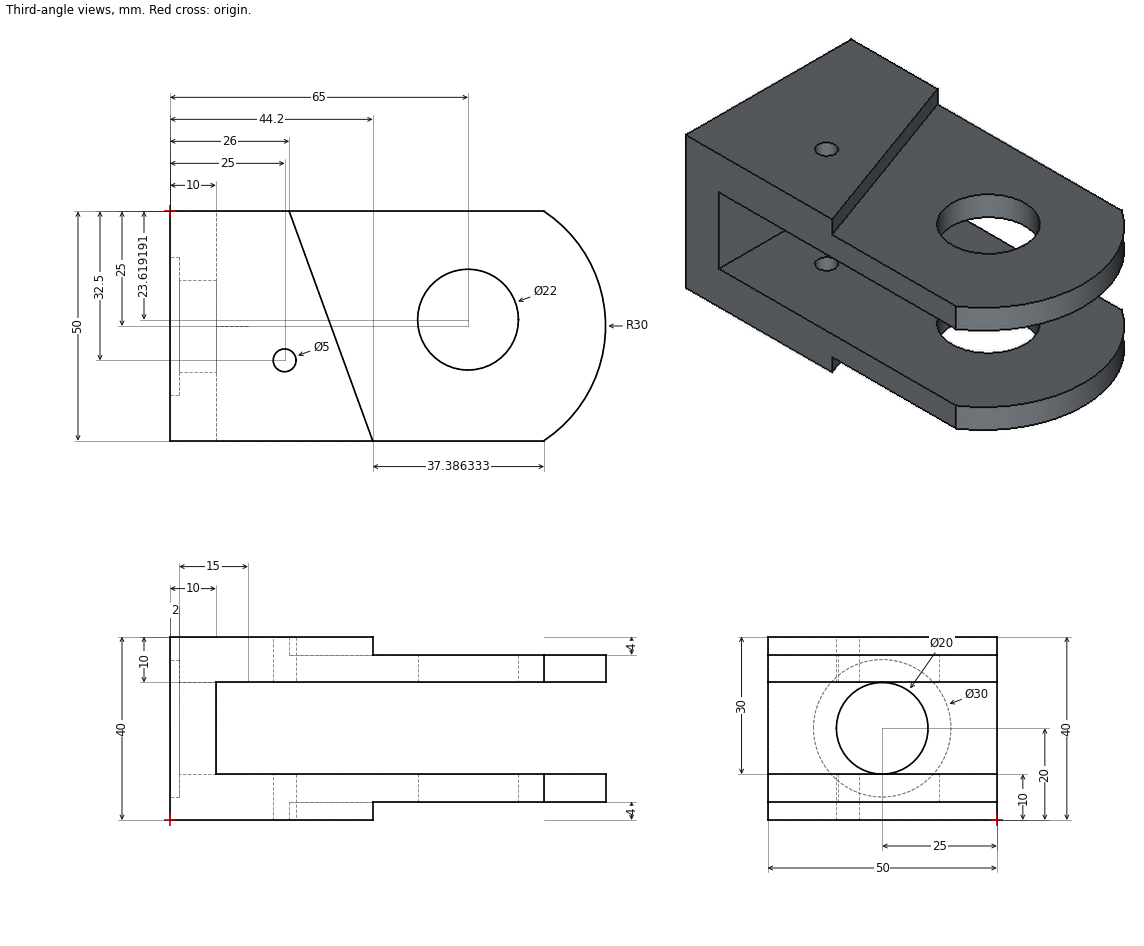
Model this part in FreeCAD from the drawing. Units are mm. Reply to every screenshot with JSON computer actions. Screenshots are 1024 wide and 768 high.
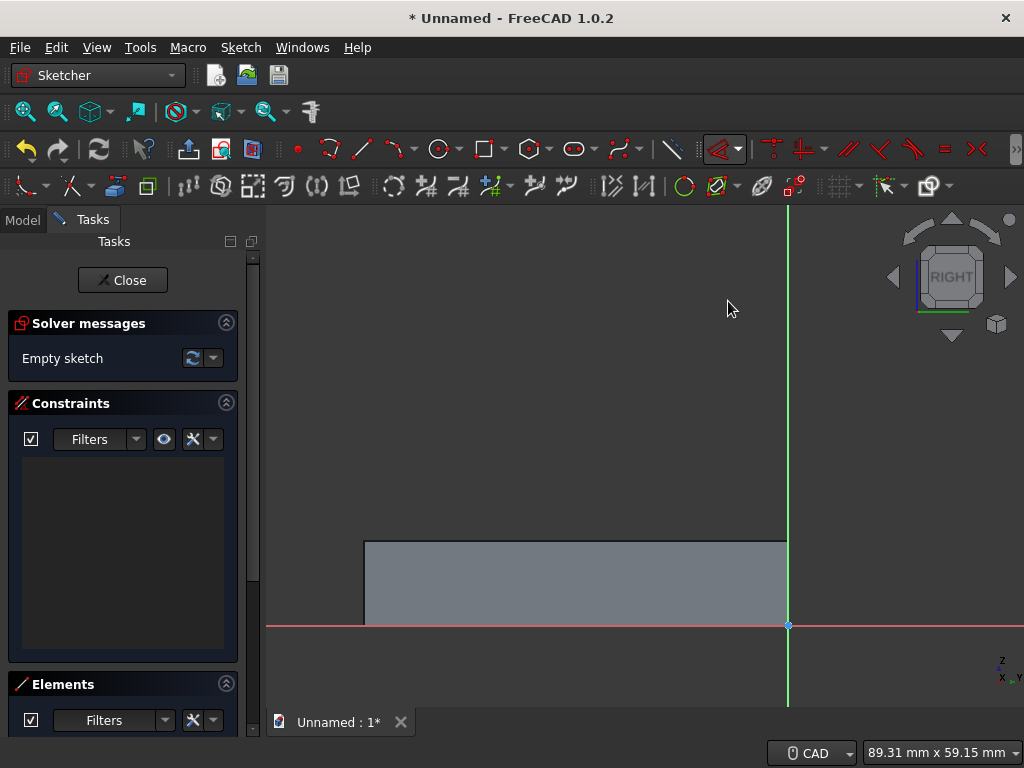
{"action": "left_click", "coordinate": [484, 150]}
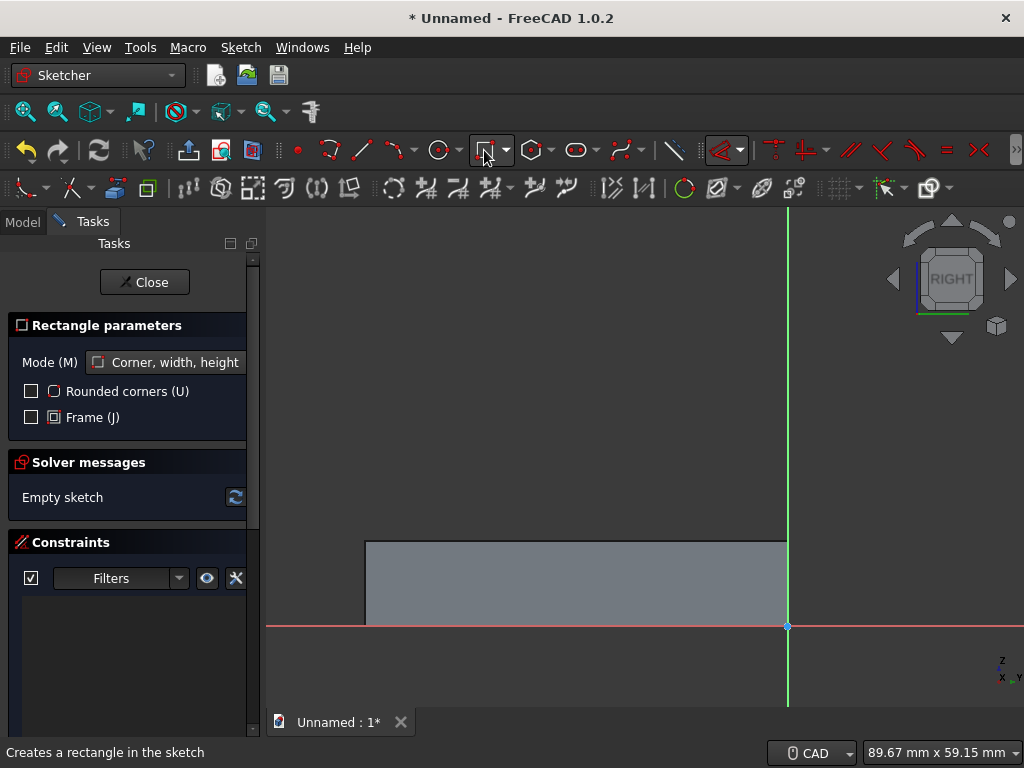
{"action": "left_click", "coordinate": [365, 288]}
{"action": "left_click", "coordinate": [788, 541]}
{"action": "key", "text": "Escape"}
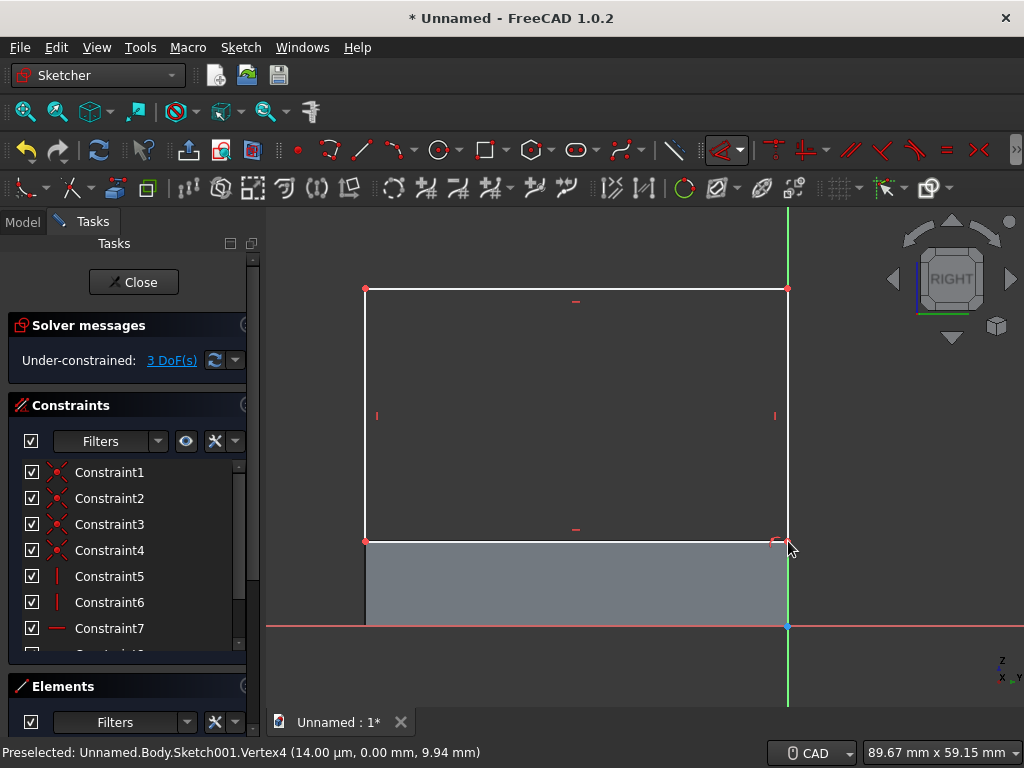
{"action": "left_click", "coordinate": [365, 365]}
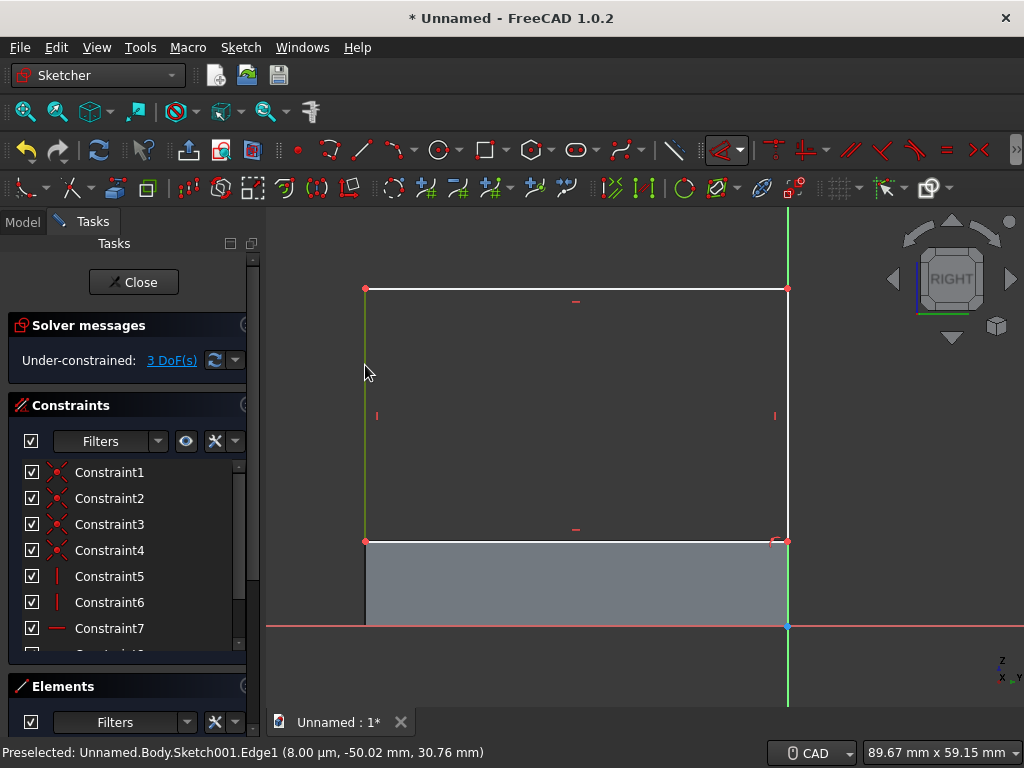
{"action": "key", "text": "i"}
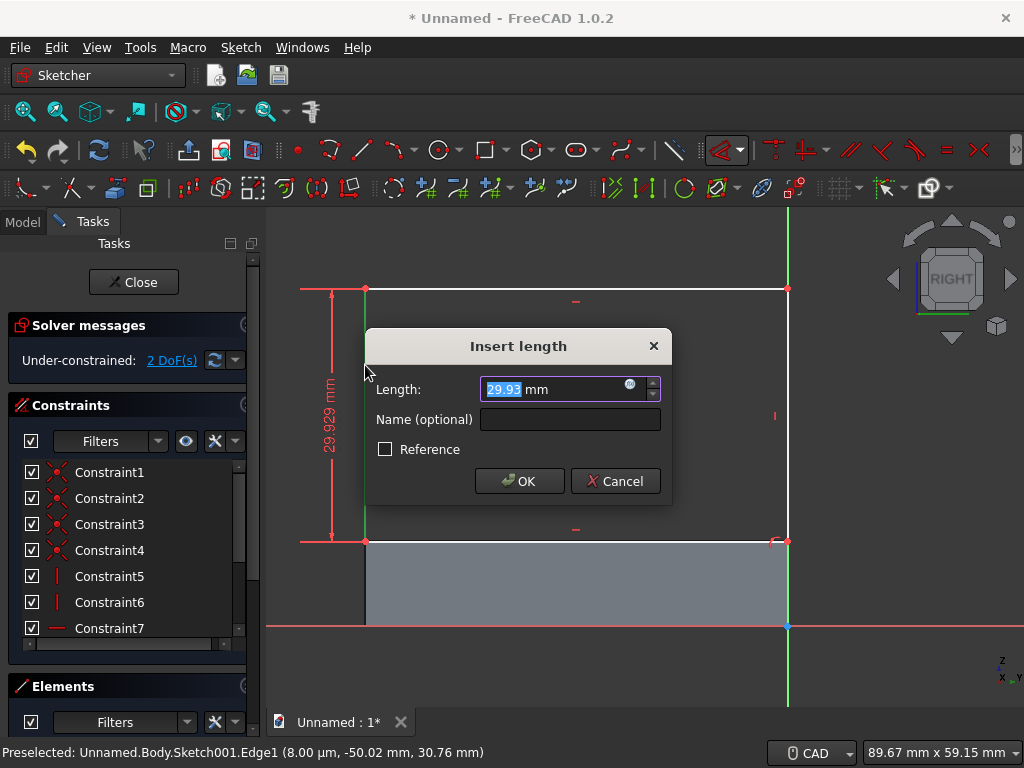
{"action": "type", "text": "30"}
{"action": "key", "text": "Return"}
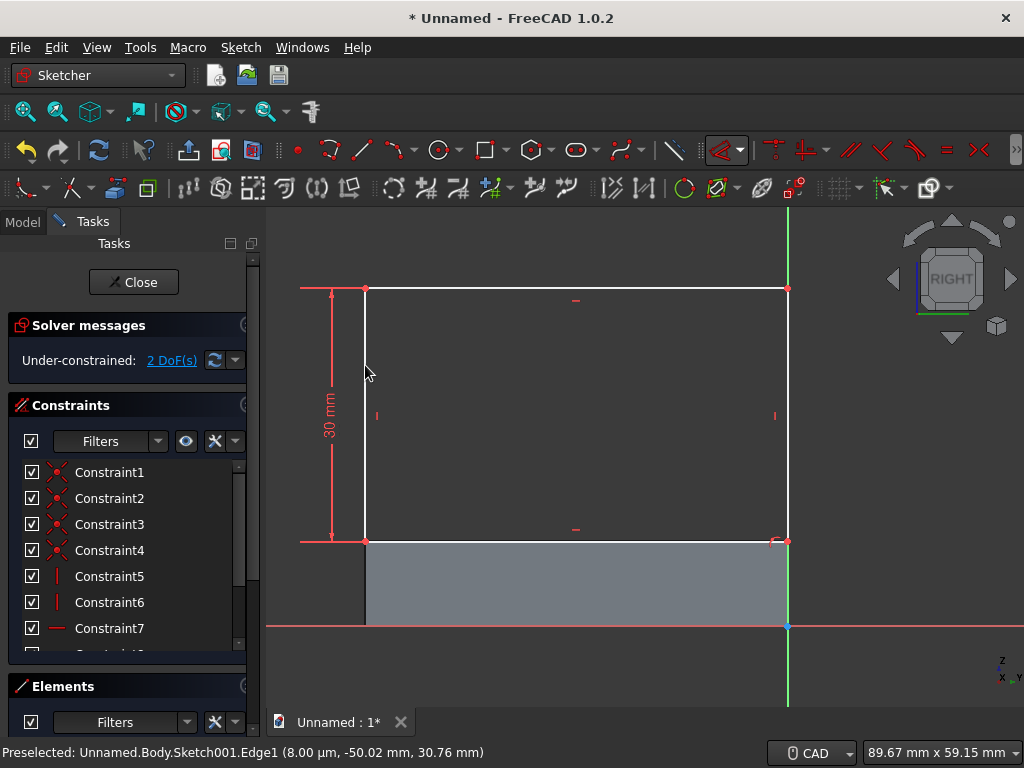
{"action": "left_click", "coordinate": [492, 542]}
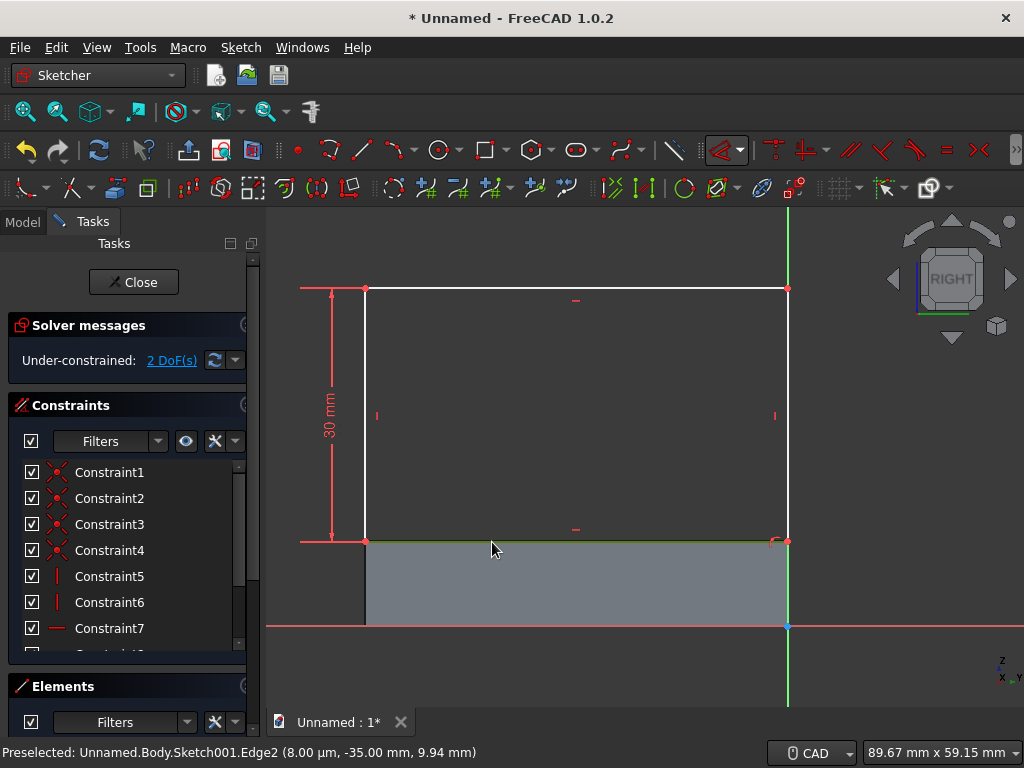
{"action": "left_click", "coordinate": [742, 150]}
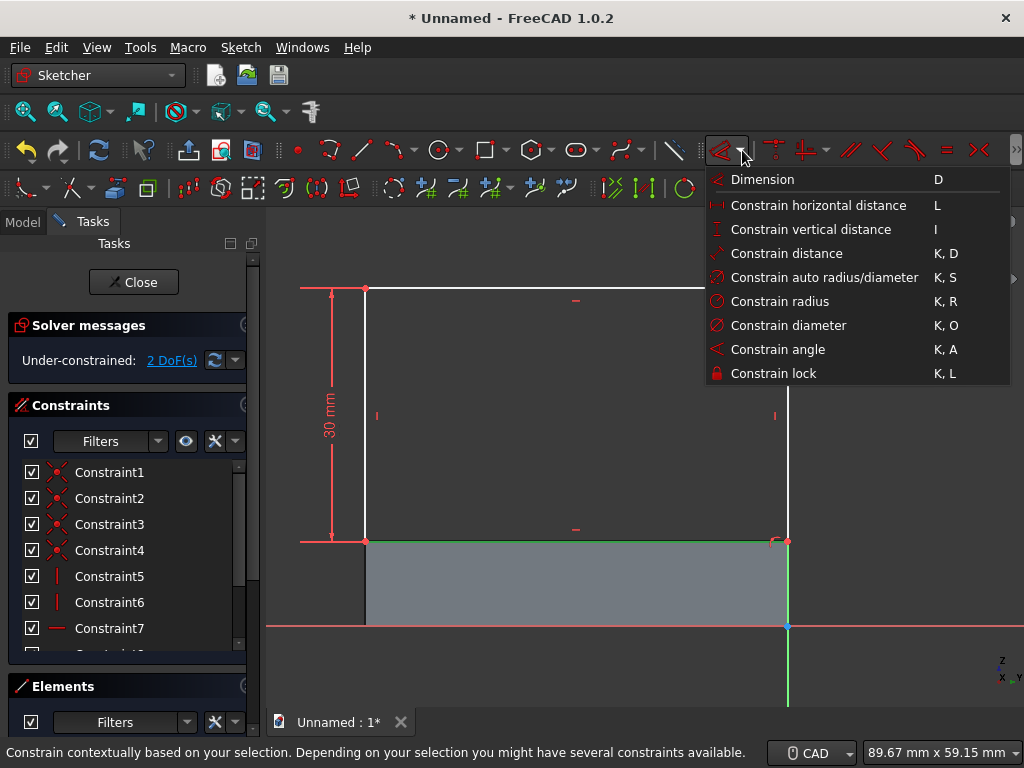
{"action": "left_click", "coordinate": [858, 205]}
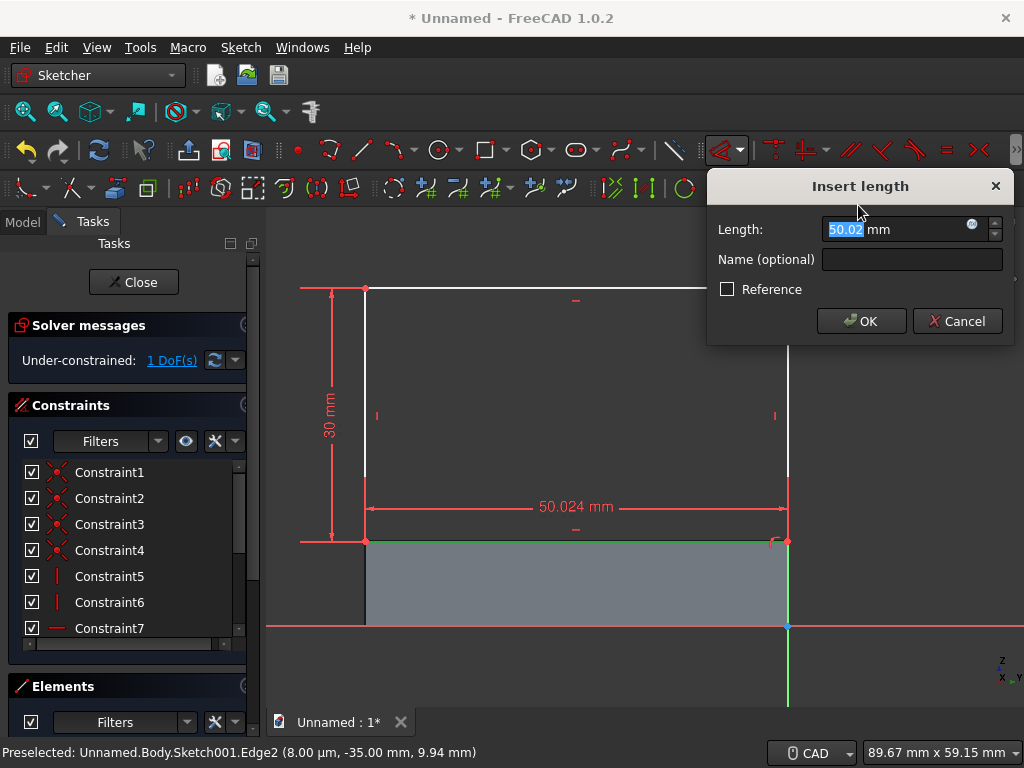
{"action": "type", "text": "50"}
{"action": "key", "text": "Return"}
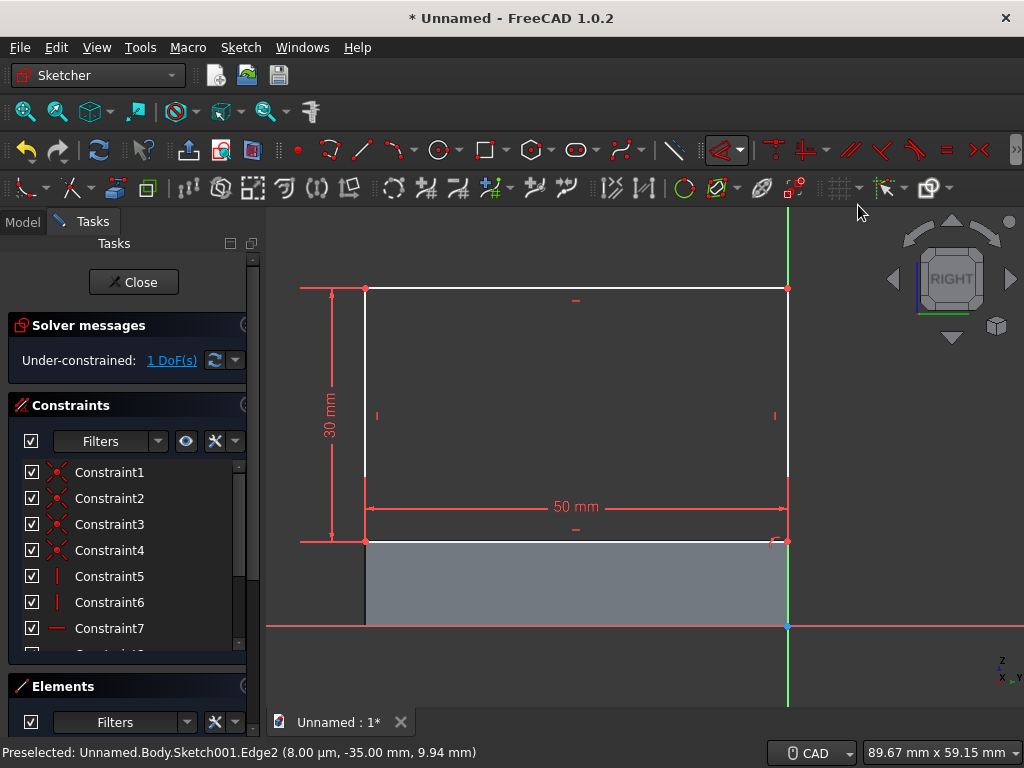
{"action": "left_click", "coordinate": [365, 288]}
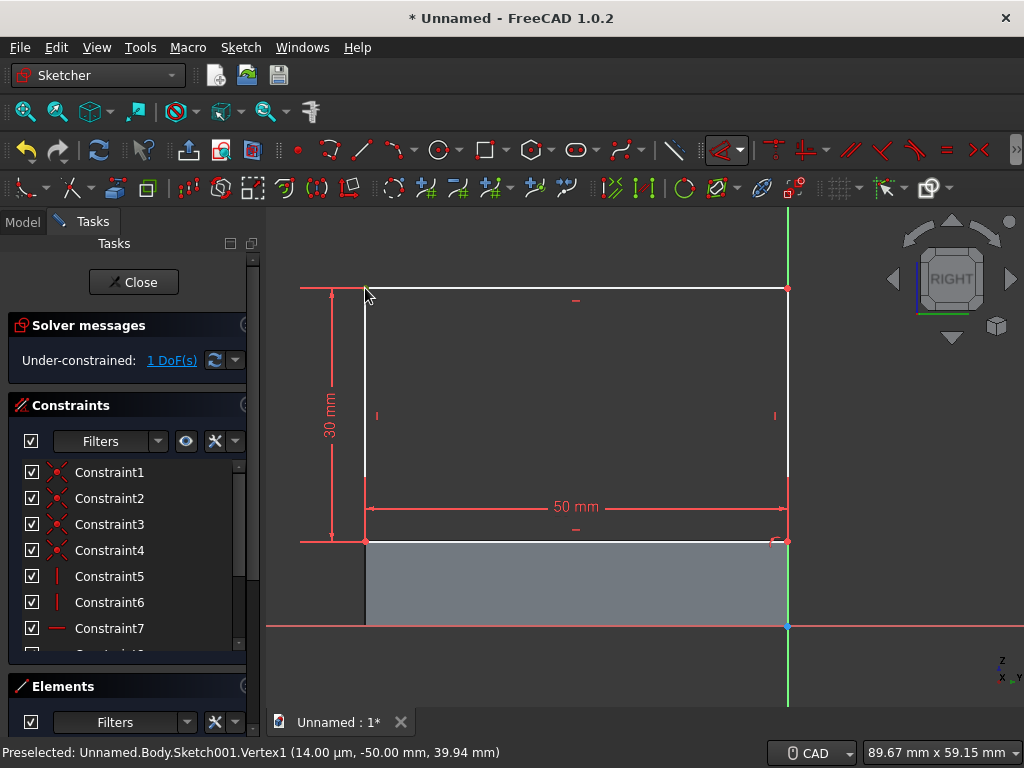
{"action": "key", "text": "i"}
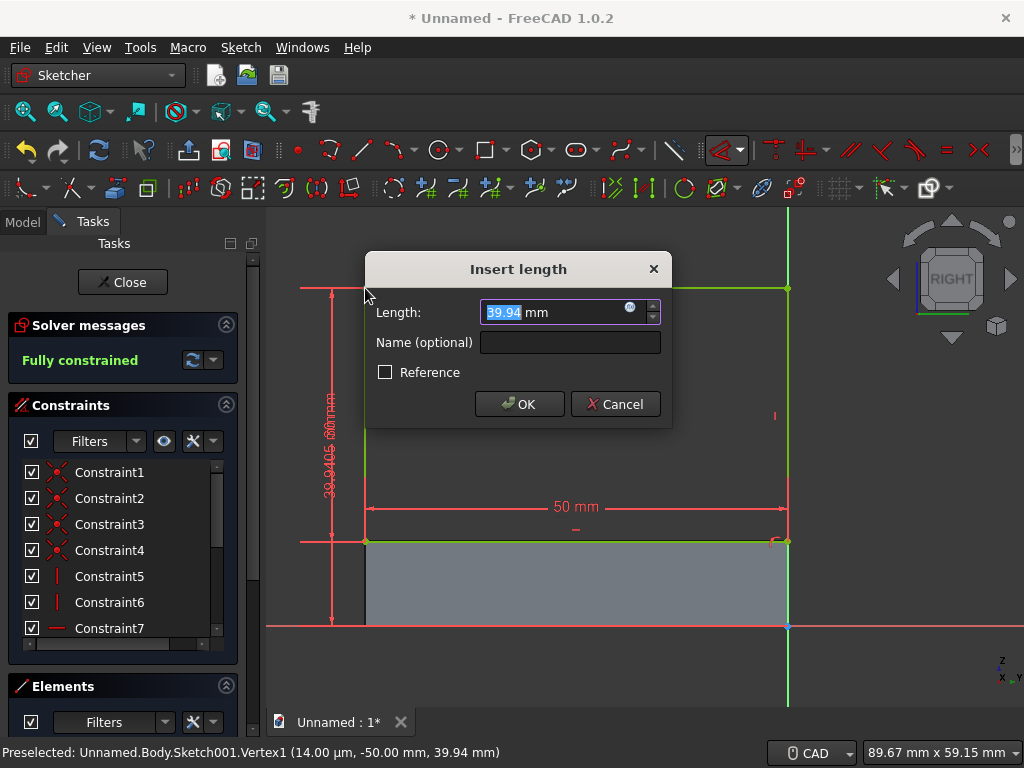
{"action": "type", "text": "40"}
{"action": "key", "text": "Return"}